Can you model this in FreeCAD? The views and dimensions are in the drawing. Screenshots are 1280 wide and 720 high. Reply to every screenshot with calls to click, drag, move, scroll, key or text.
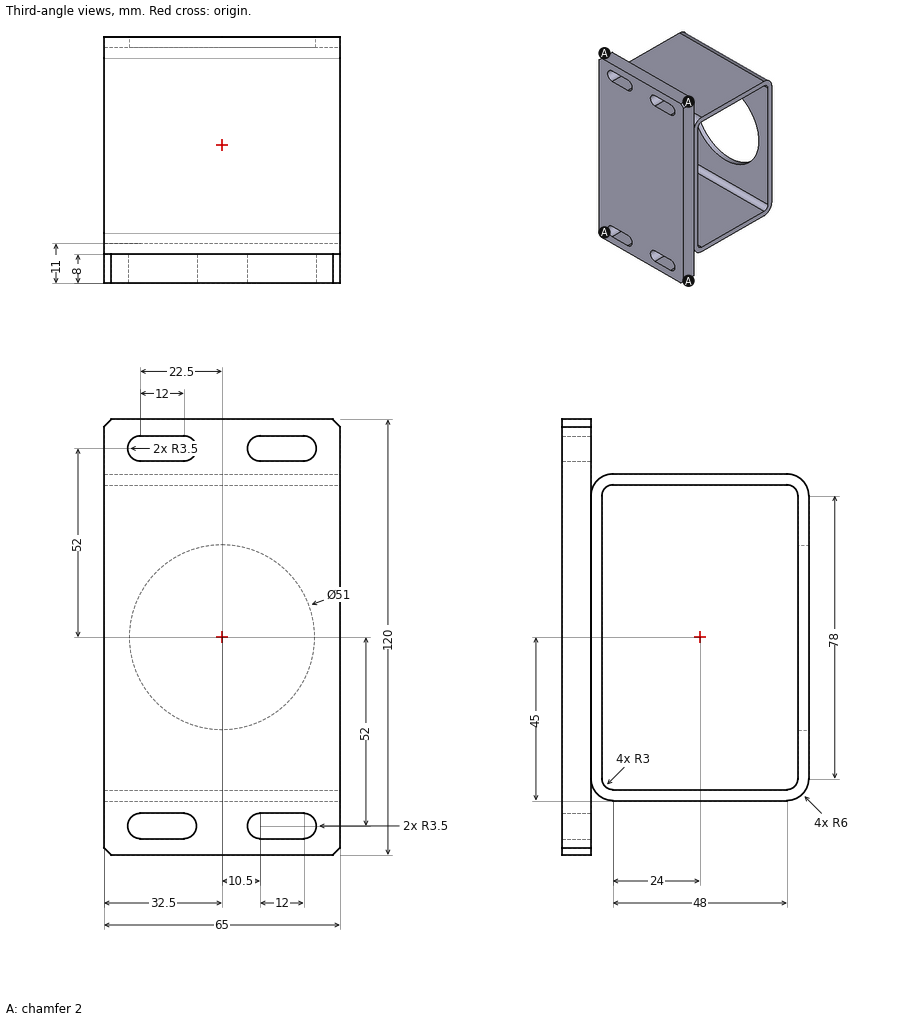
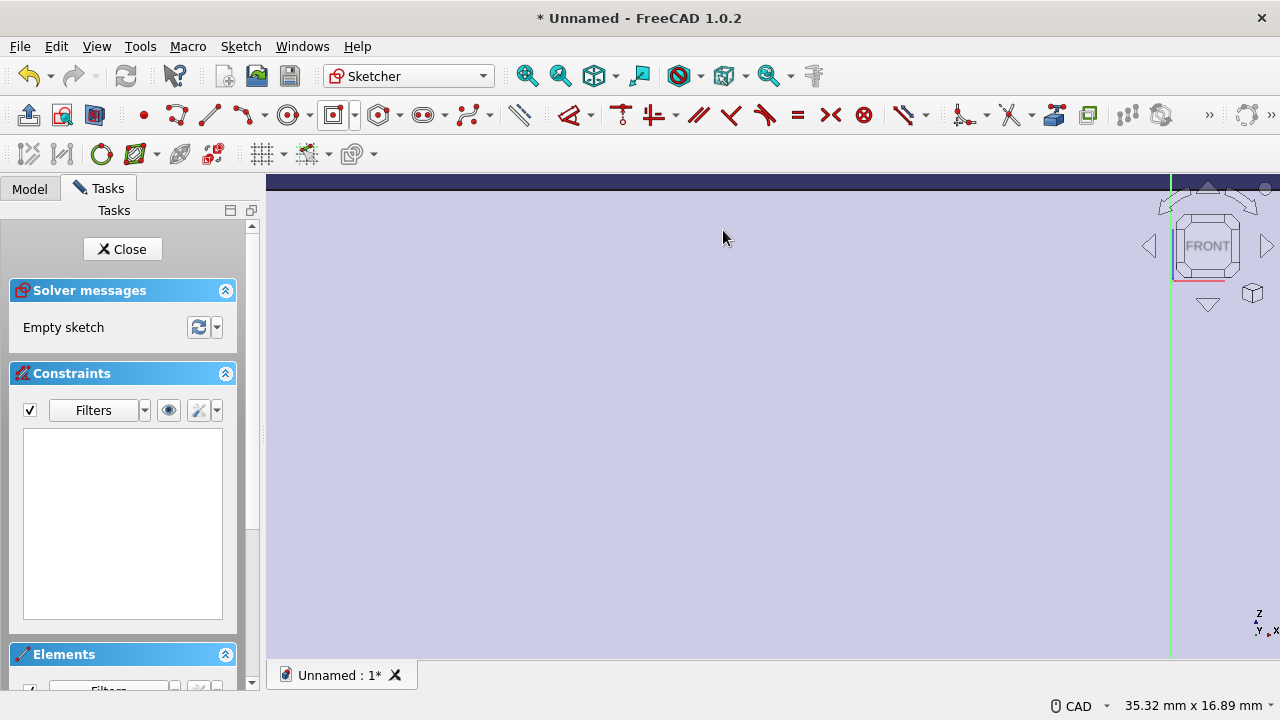
click(422, 116)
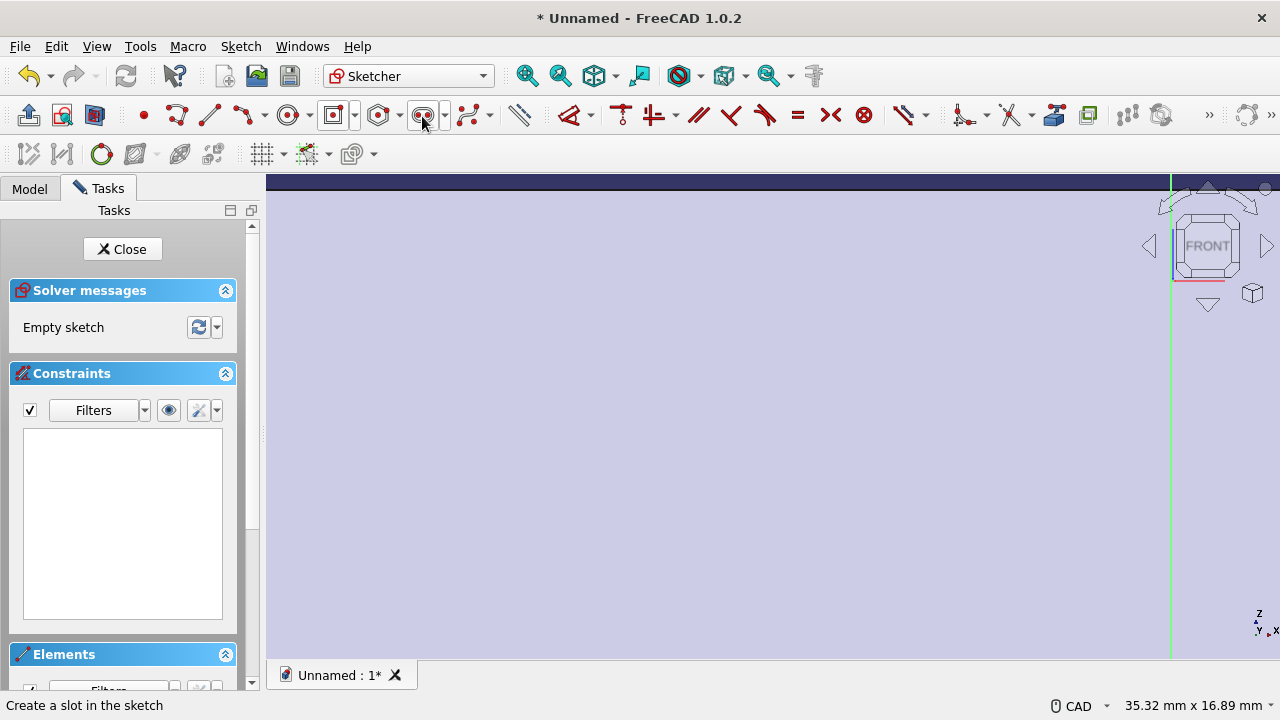
click(525, 419)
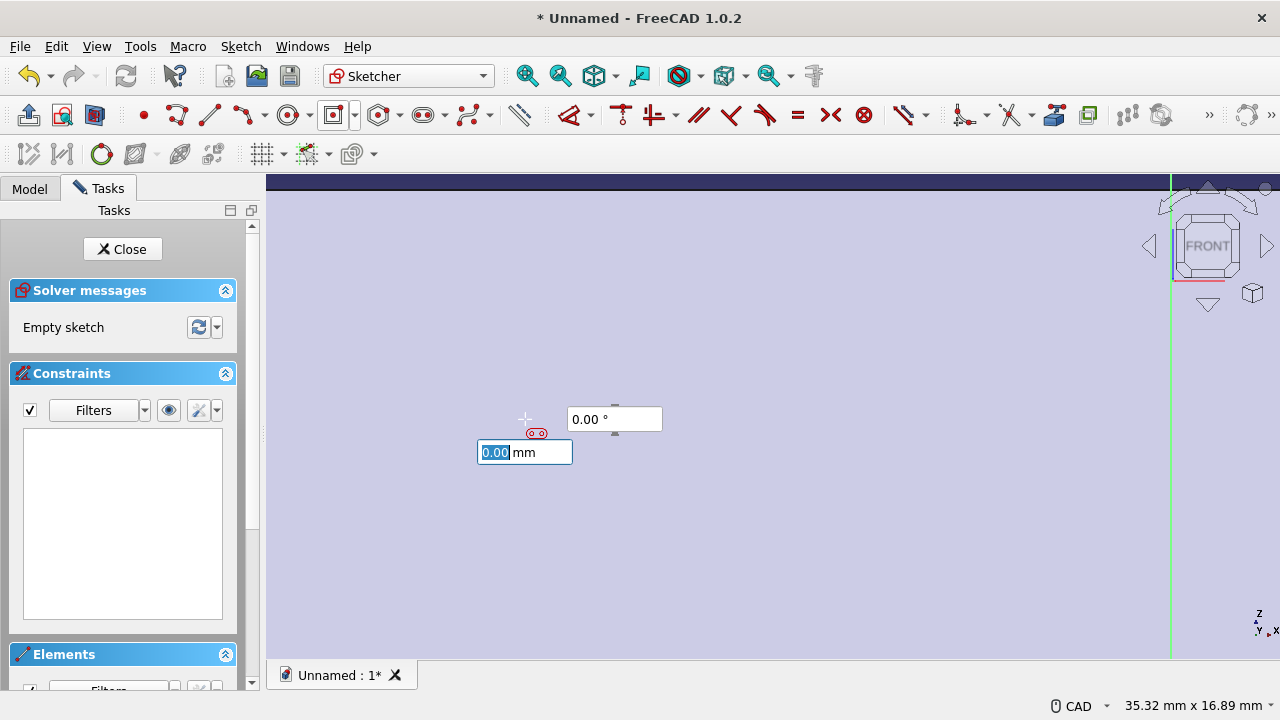
click(869, 419)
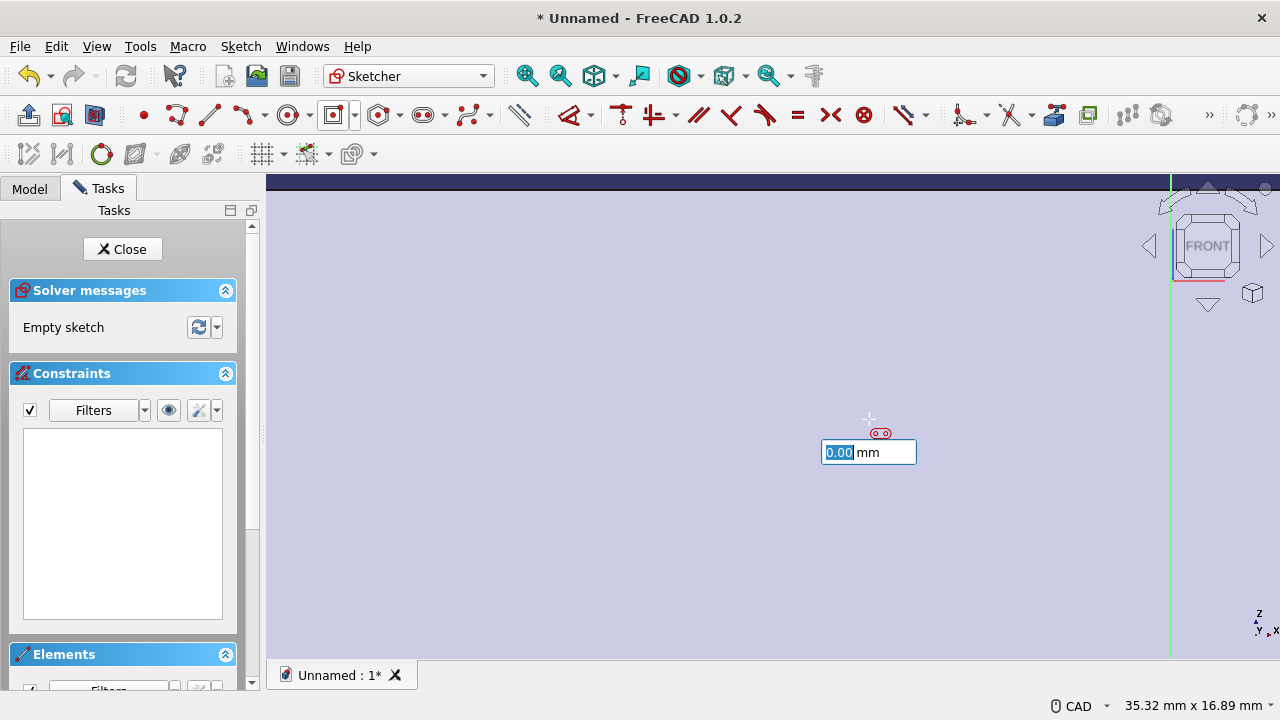
click(697, 319)
key(Escape)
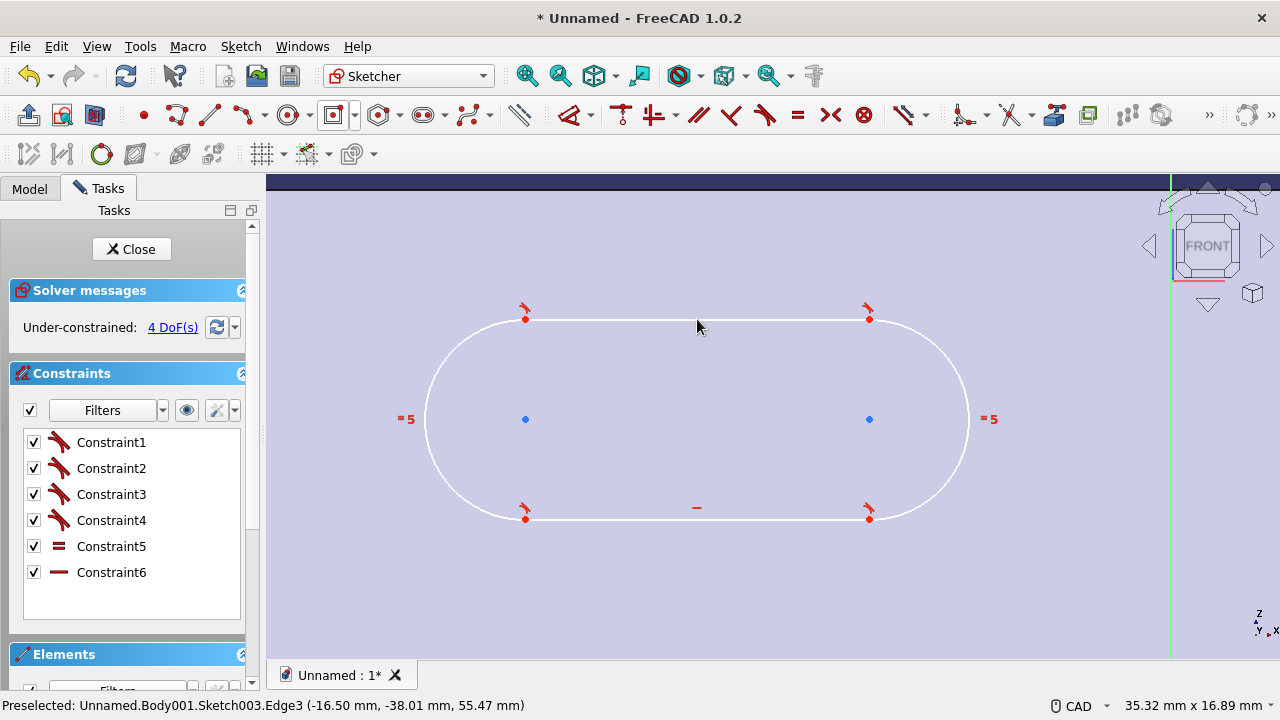
click(568, 116)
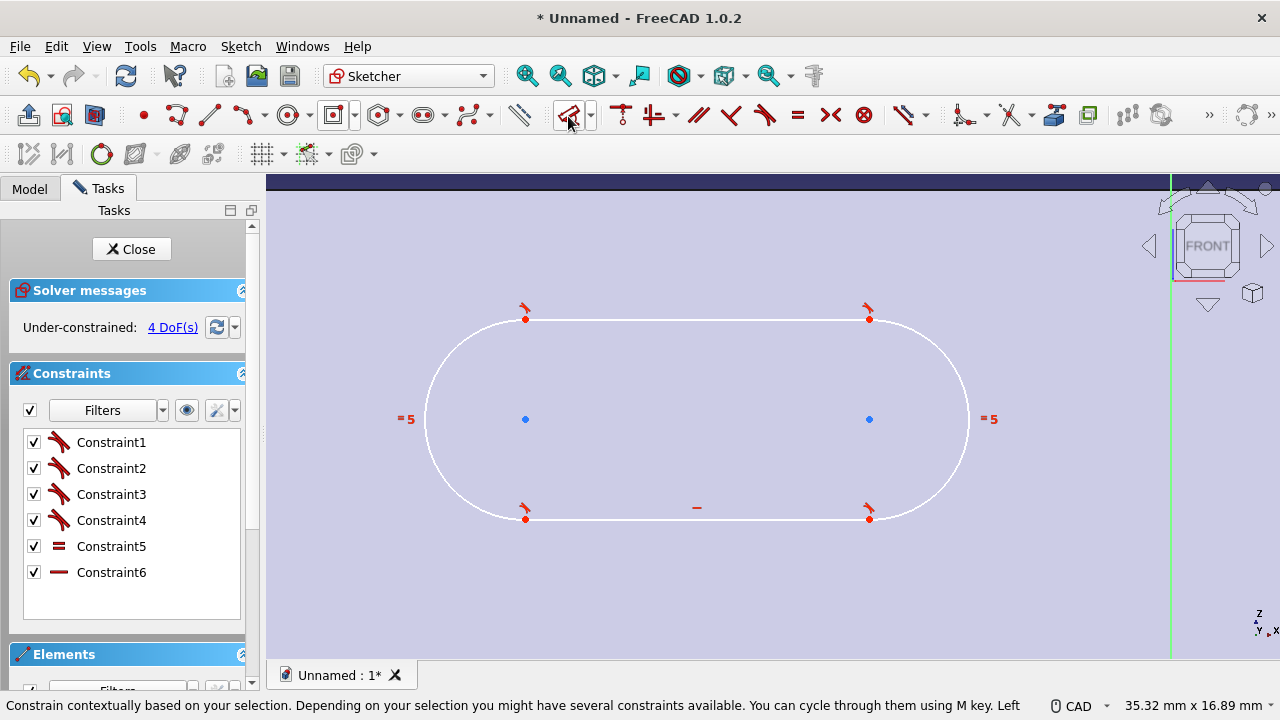
click(444, 361)
click(418, 342)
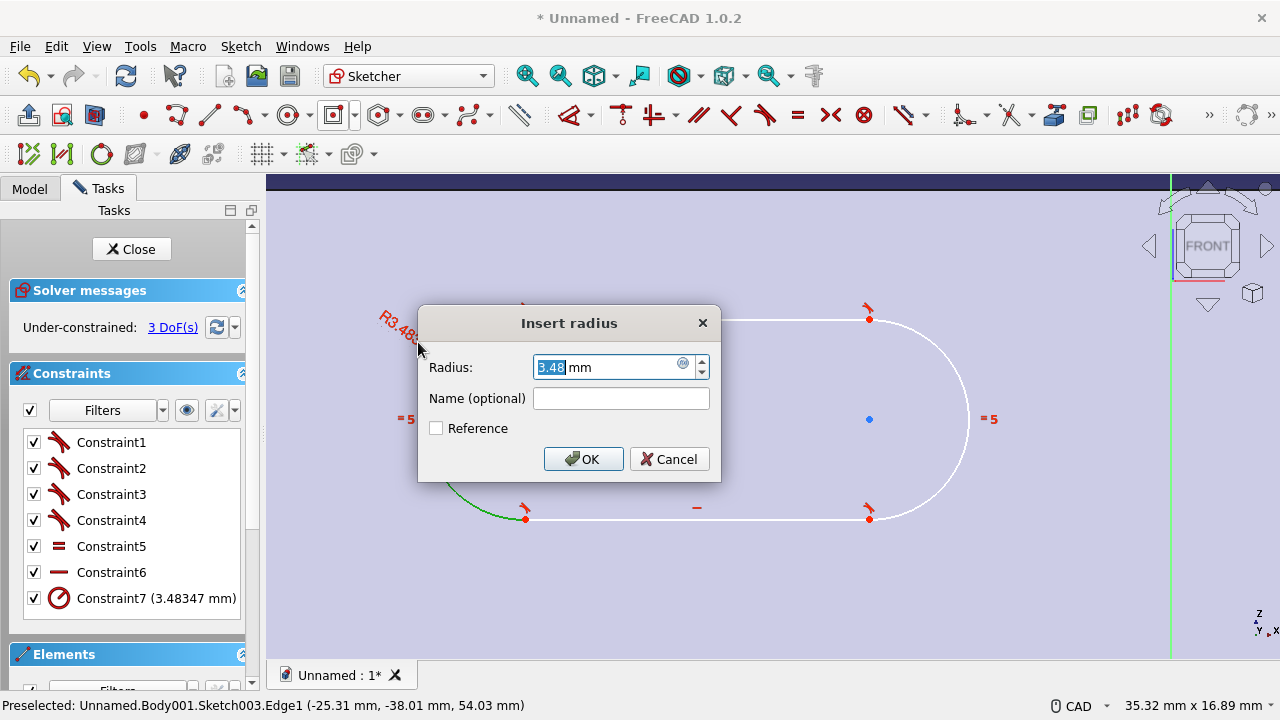
text(3.5)
key(Return)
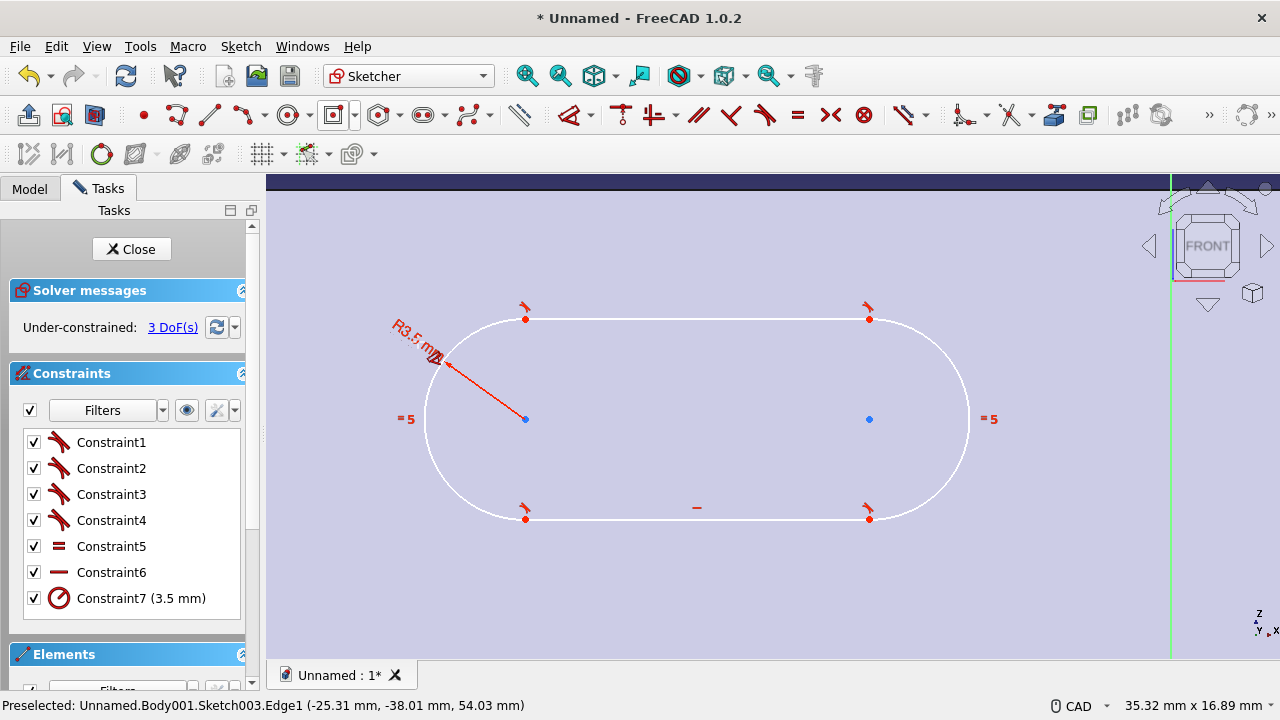
click(628, 319)
click(697, 285)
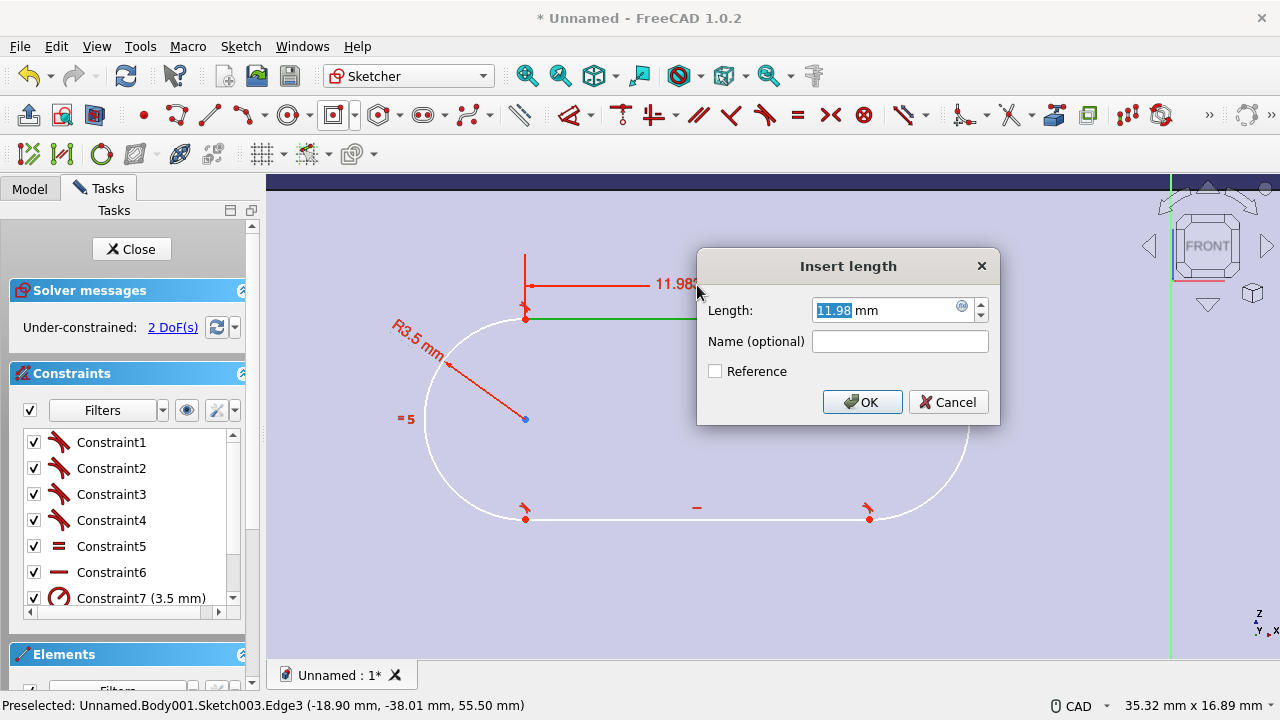
text(12)
key(Return)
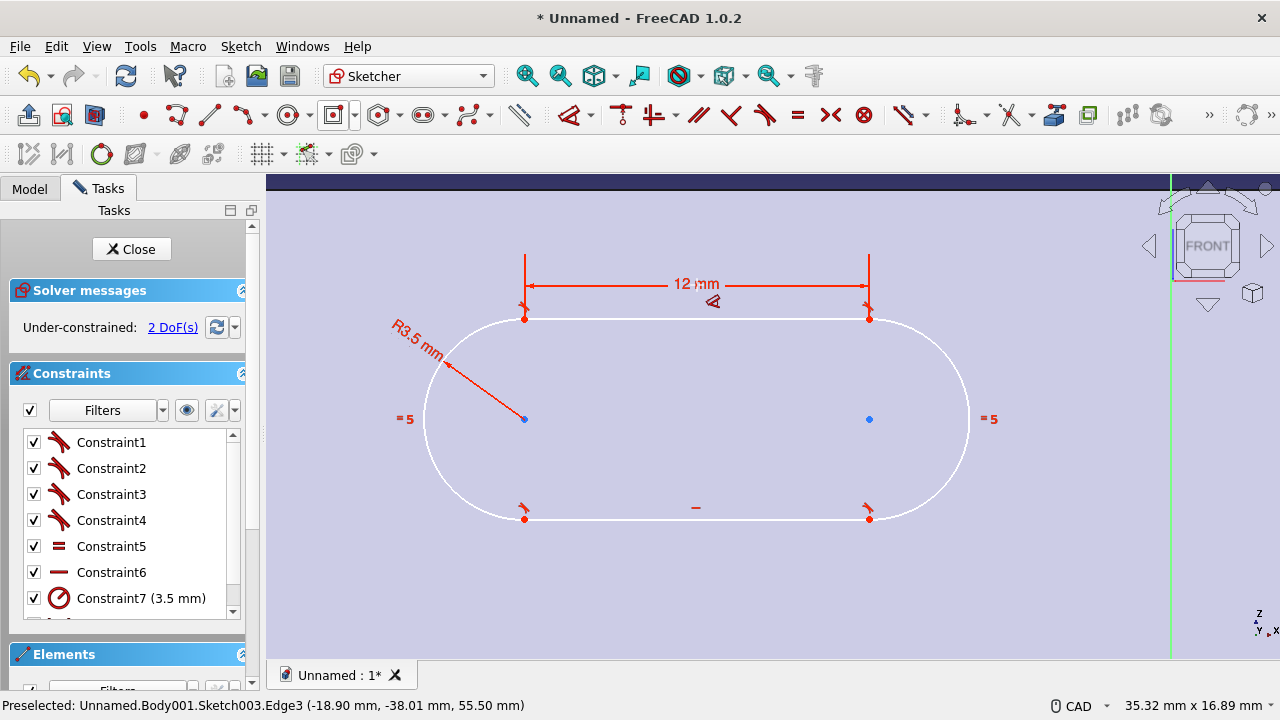
click(525, 420)
click(491, 477)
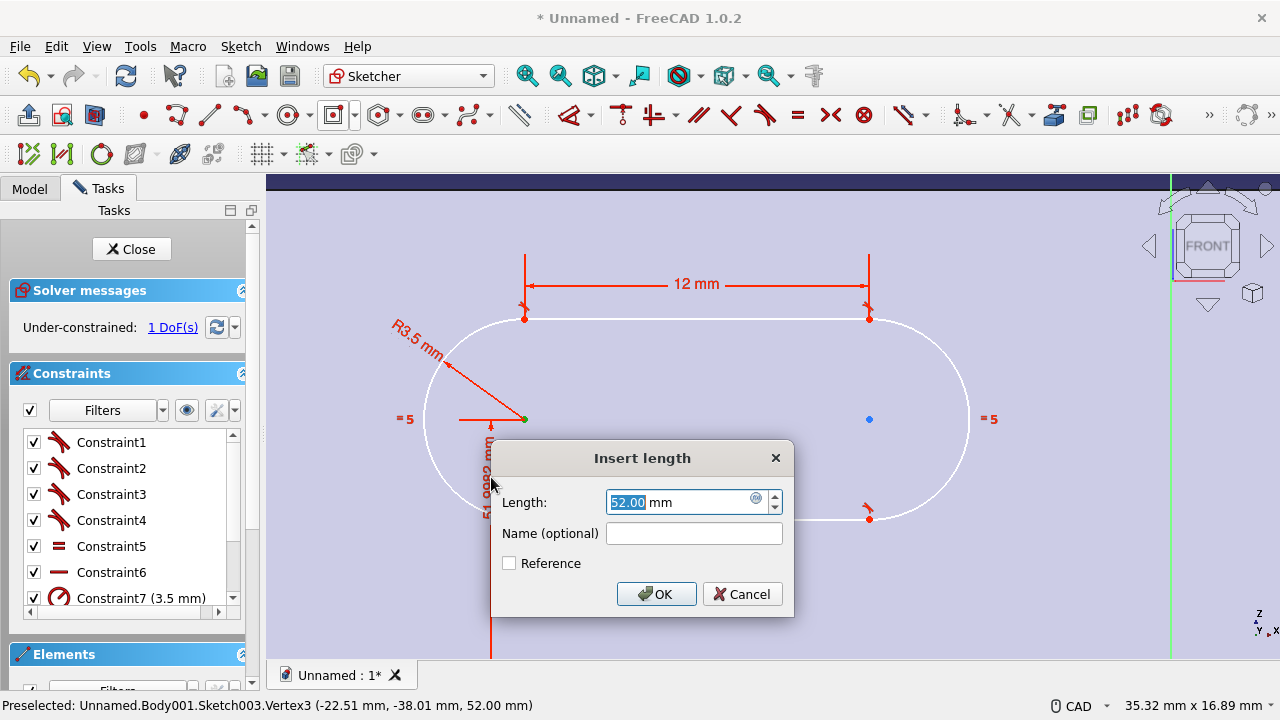
text(52)
key(Return)